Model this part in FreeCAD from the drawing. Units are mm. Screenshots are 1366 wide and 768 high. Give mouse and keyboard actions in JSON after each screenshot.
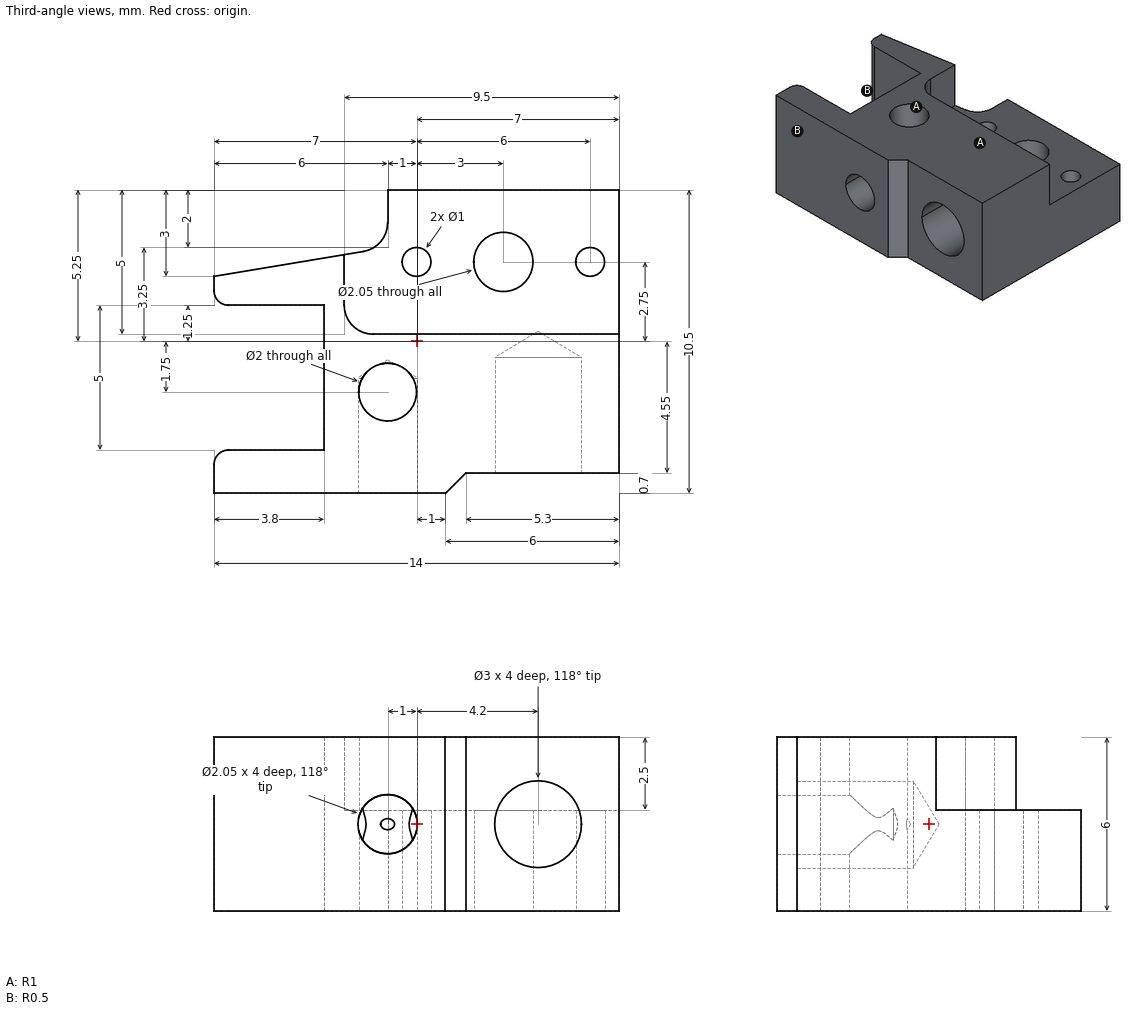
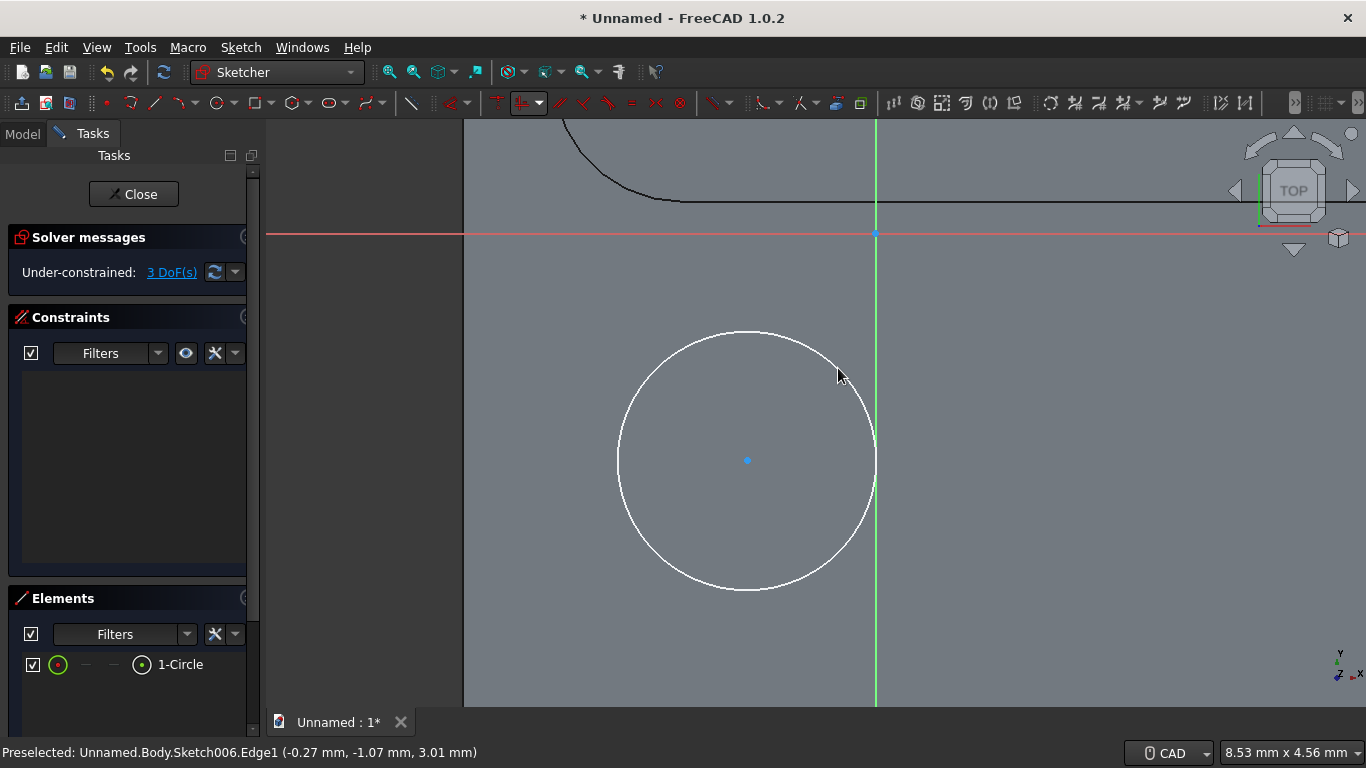
{"action": "left_click", "coordinate": [450, 104]}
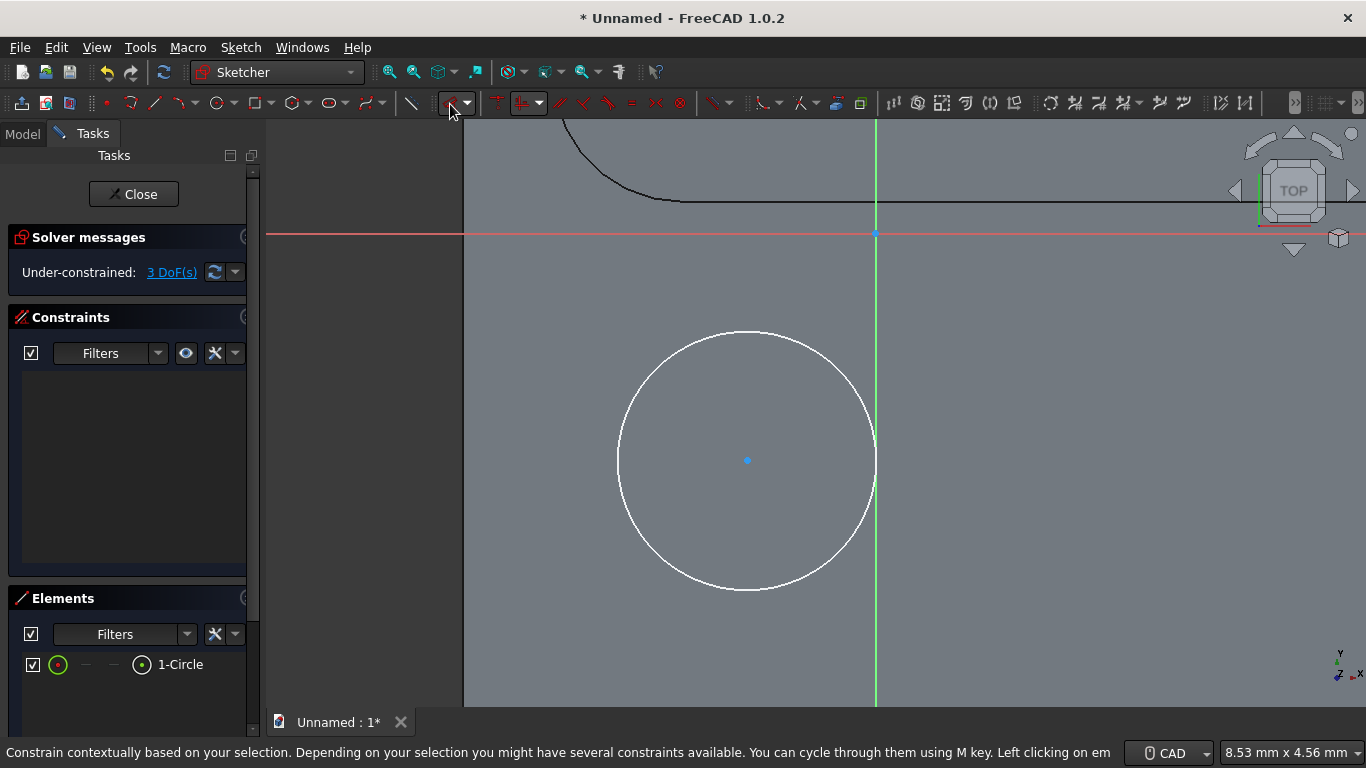
{"action": "left_click", "coordinate": [838, 369]}
{"action": "left_click", "coordinate": [861, 346]}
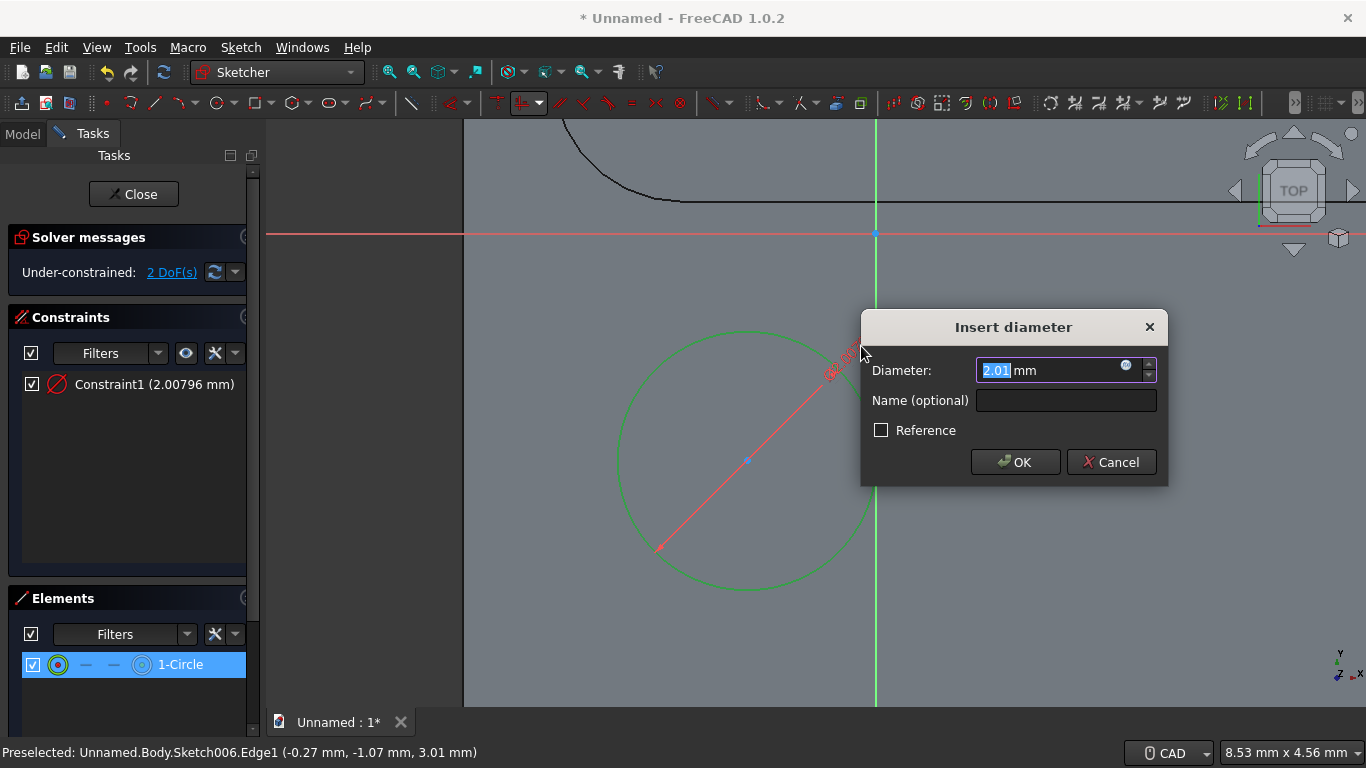
{"action": "type", "text": "2"}
{"action": "key", "text": "Return"}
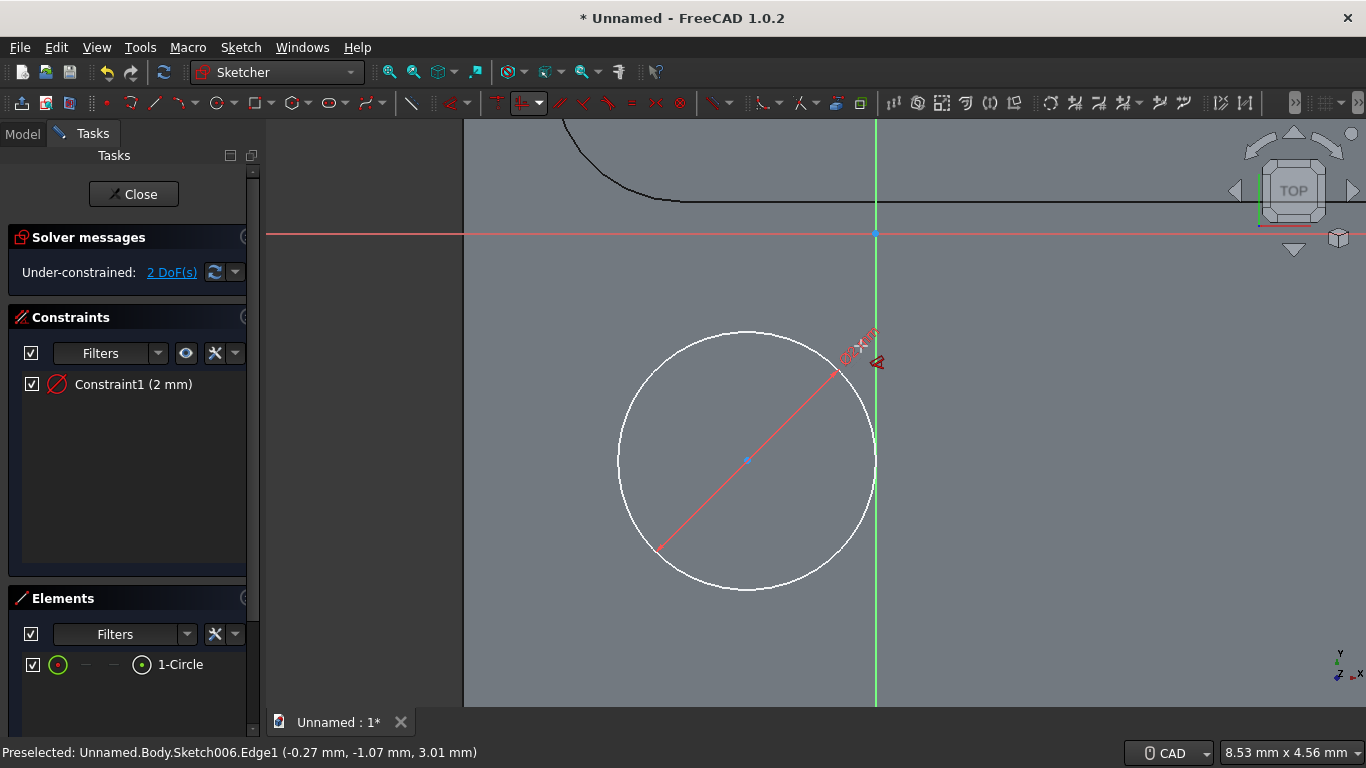
{"action": "left_click", "coordinate": [747, 461]}
{"action": "left_click", "coordinate": [811, 200]}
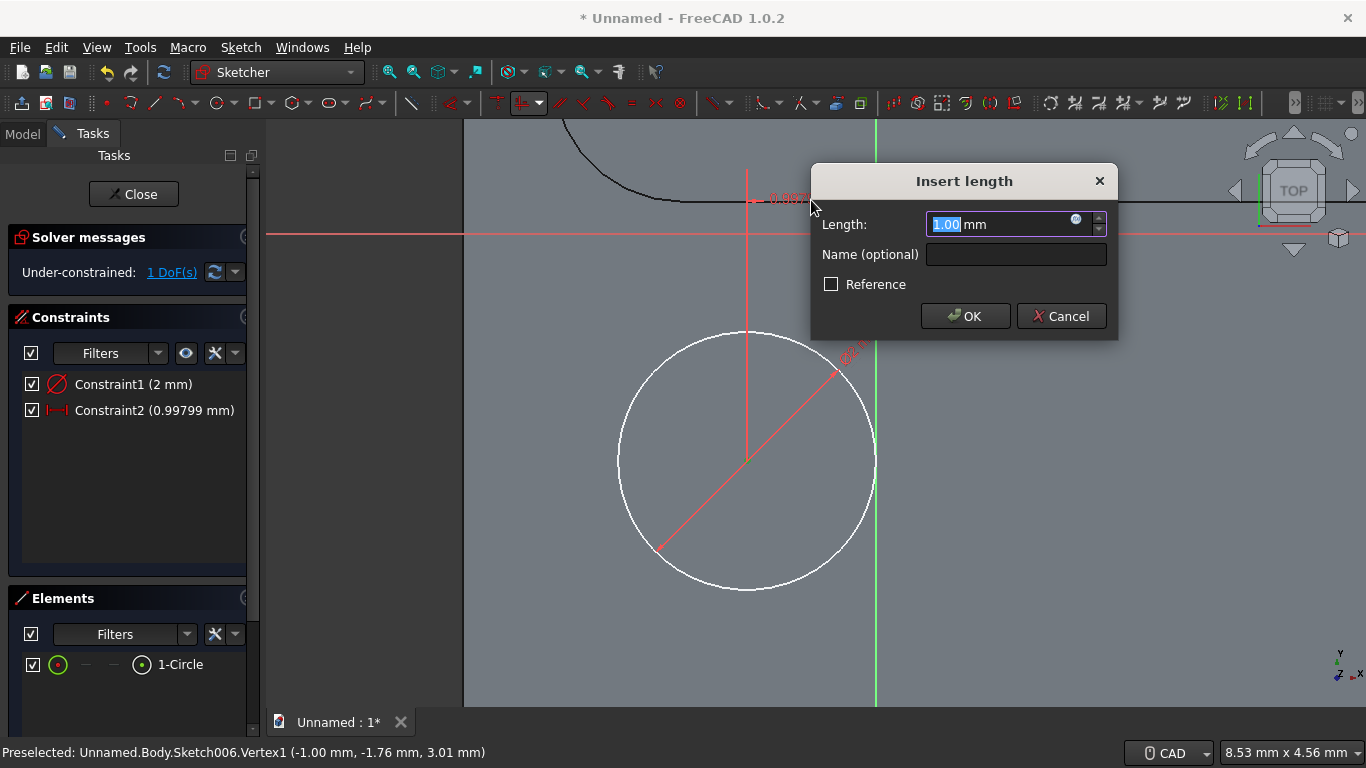
{"action": "type", "text": "1"}
{"action": "key", "text": "Return"}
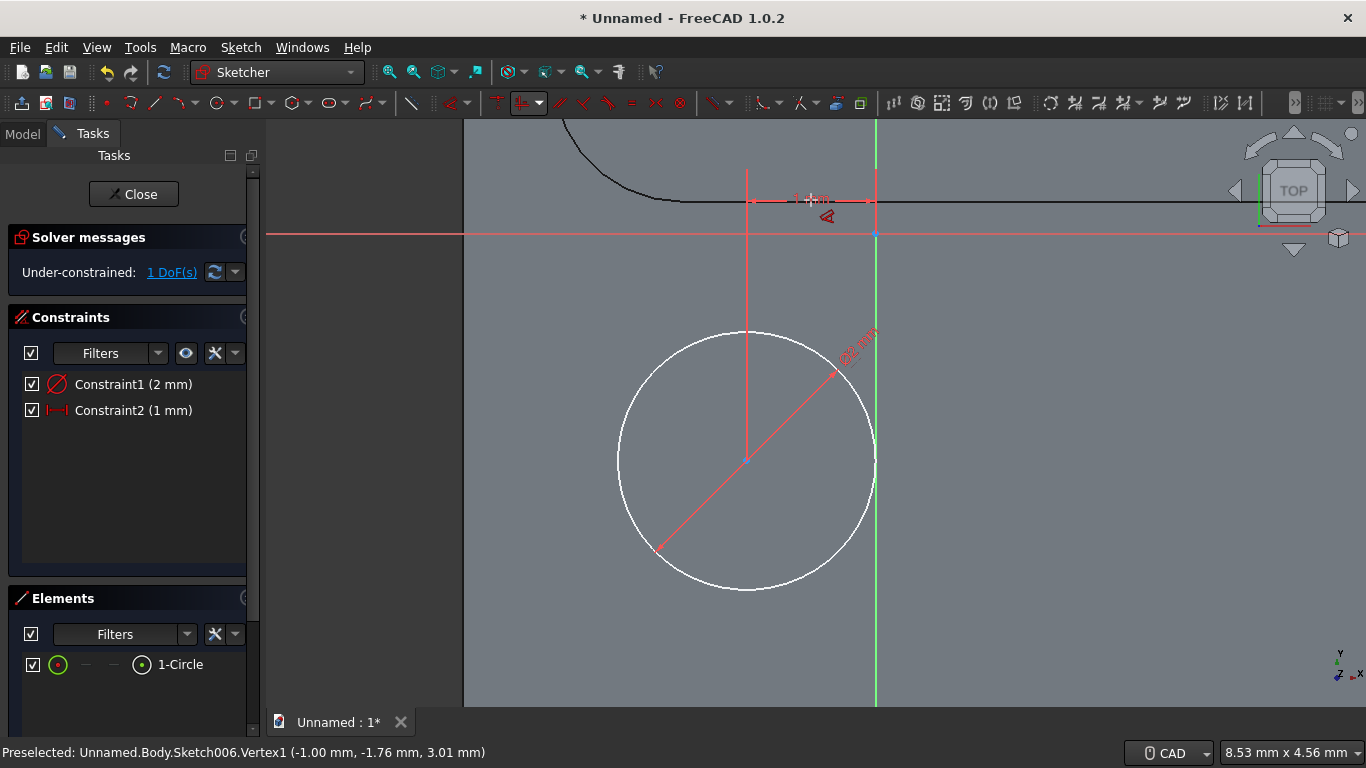
{"action": "left_click", "coordinate": [747, 461]}
{"action": "left_click", "coordinate": [910, 295]}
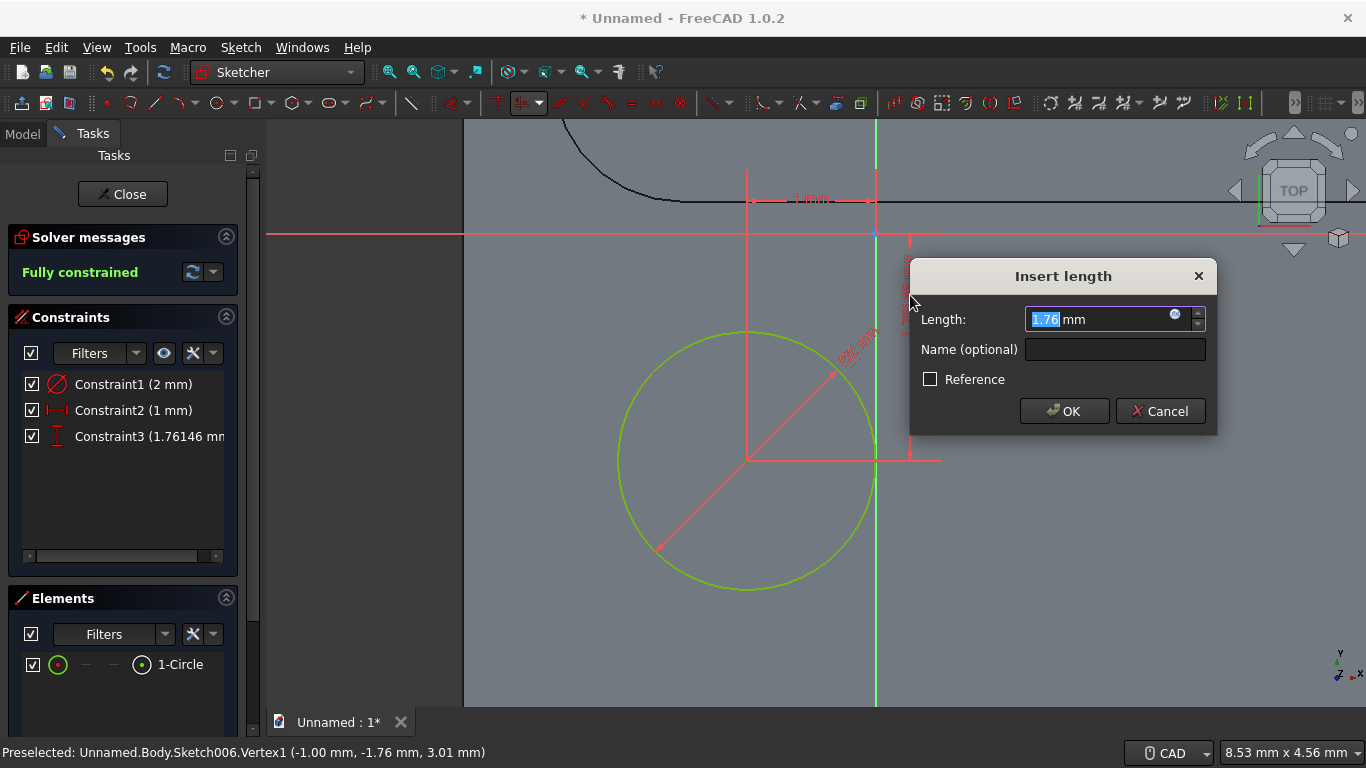
{"action": "type", "text": "1.75"}
{"action": "key", "text": "Return"}
{"action": "key", "text": "Escape"}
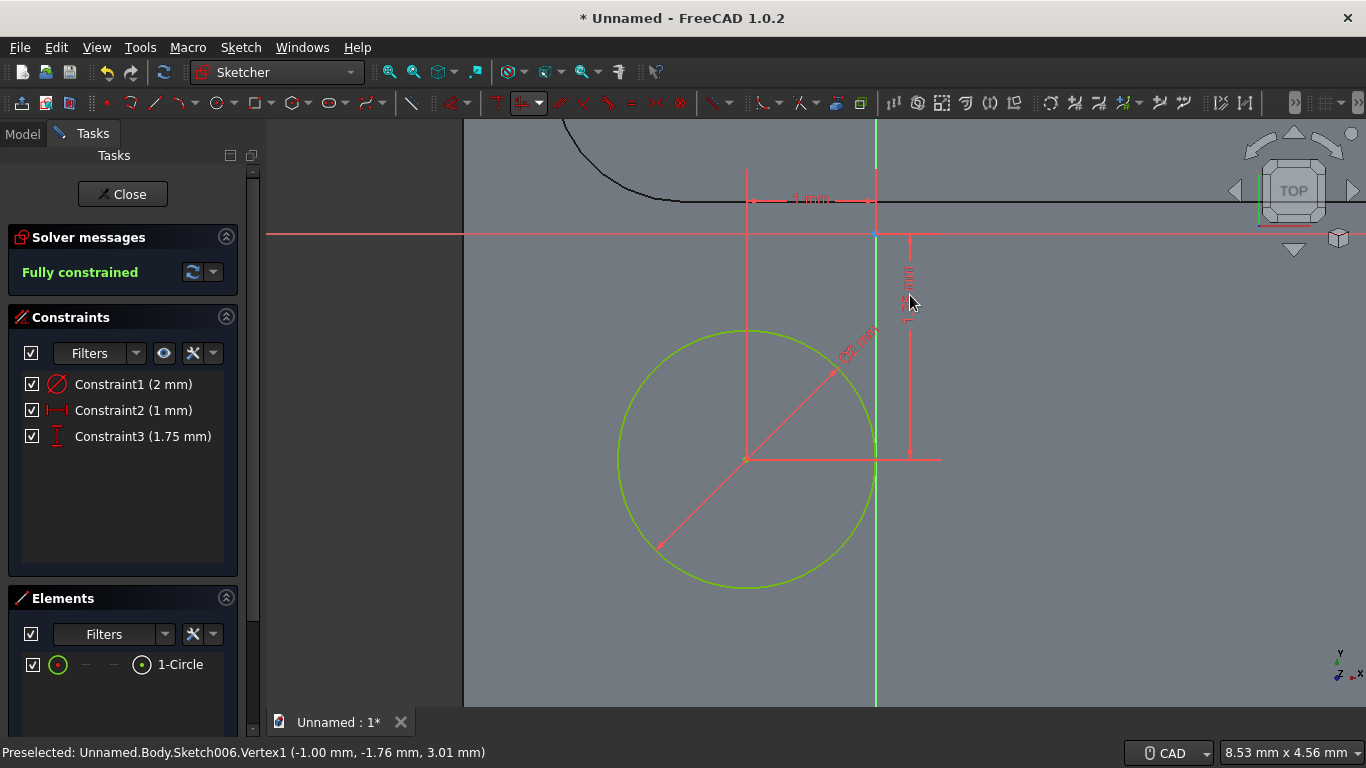
{"action": "left_click", "coordinate": [123, 194]}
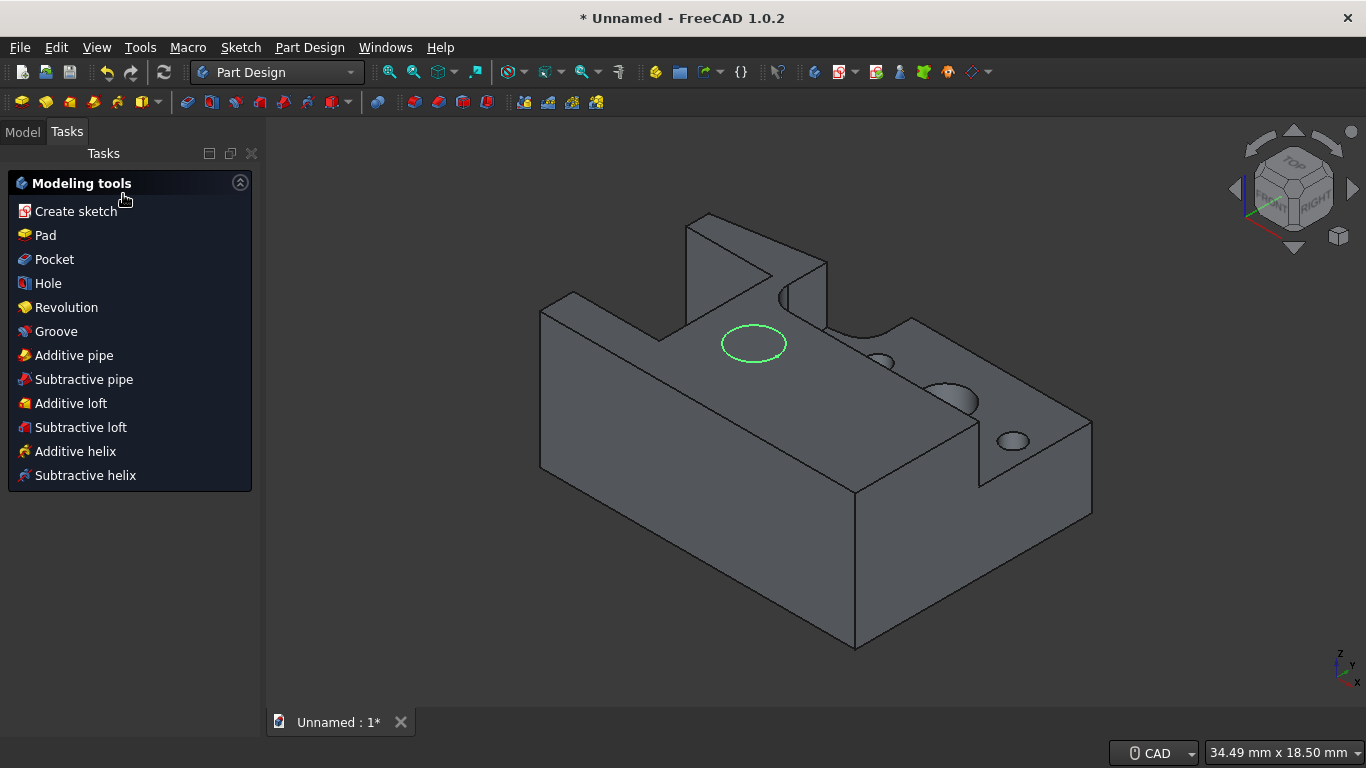
{"action": "left_click", "coordinate": [212, 102]}